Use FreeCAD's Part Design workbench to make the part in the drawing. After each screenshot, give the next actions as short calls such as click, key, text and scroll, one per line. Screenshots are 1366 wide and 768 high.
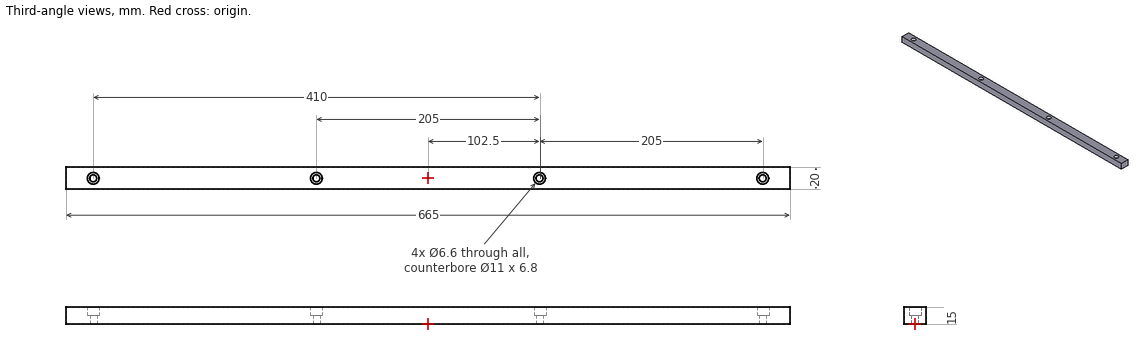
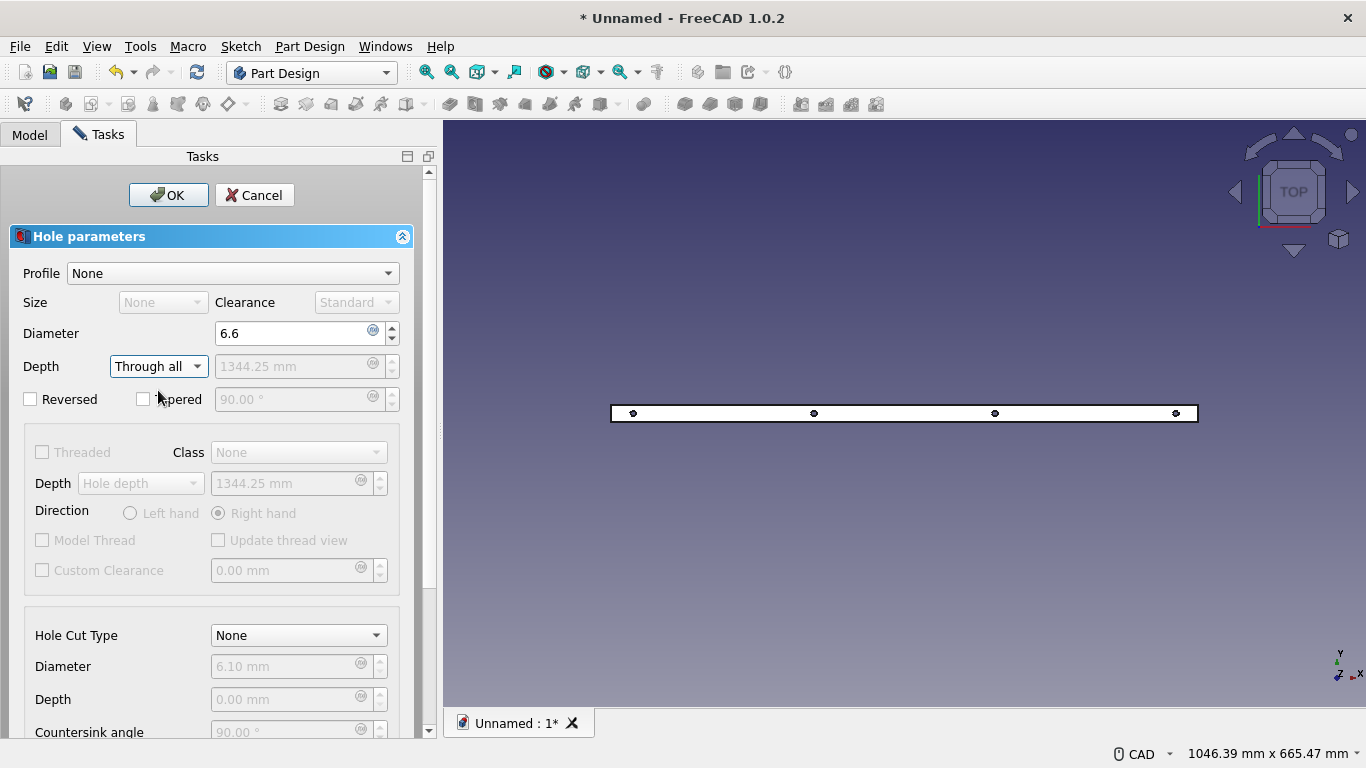
click(300, 636)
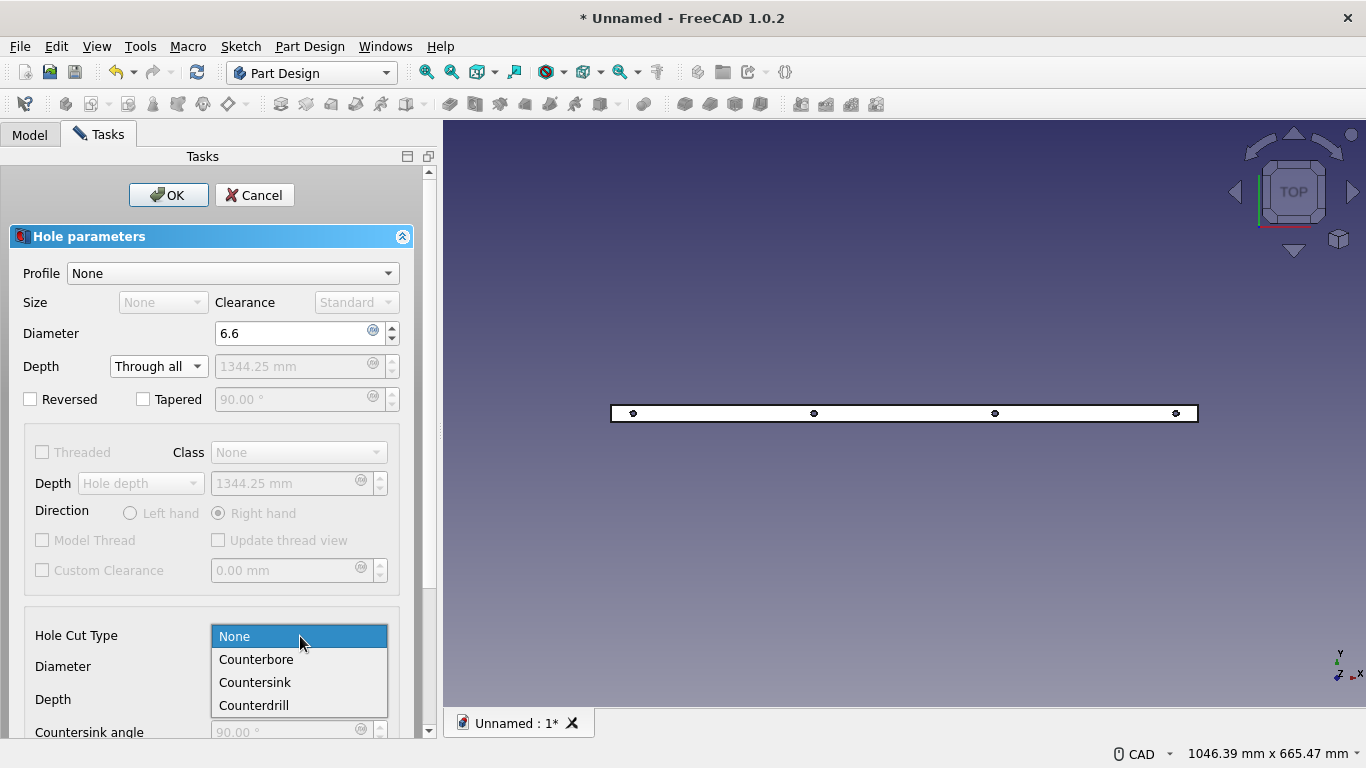
click(298, 660)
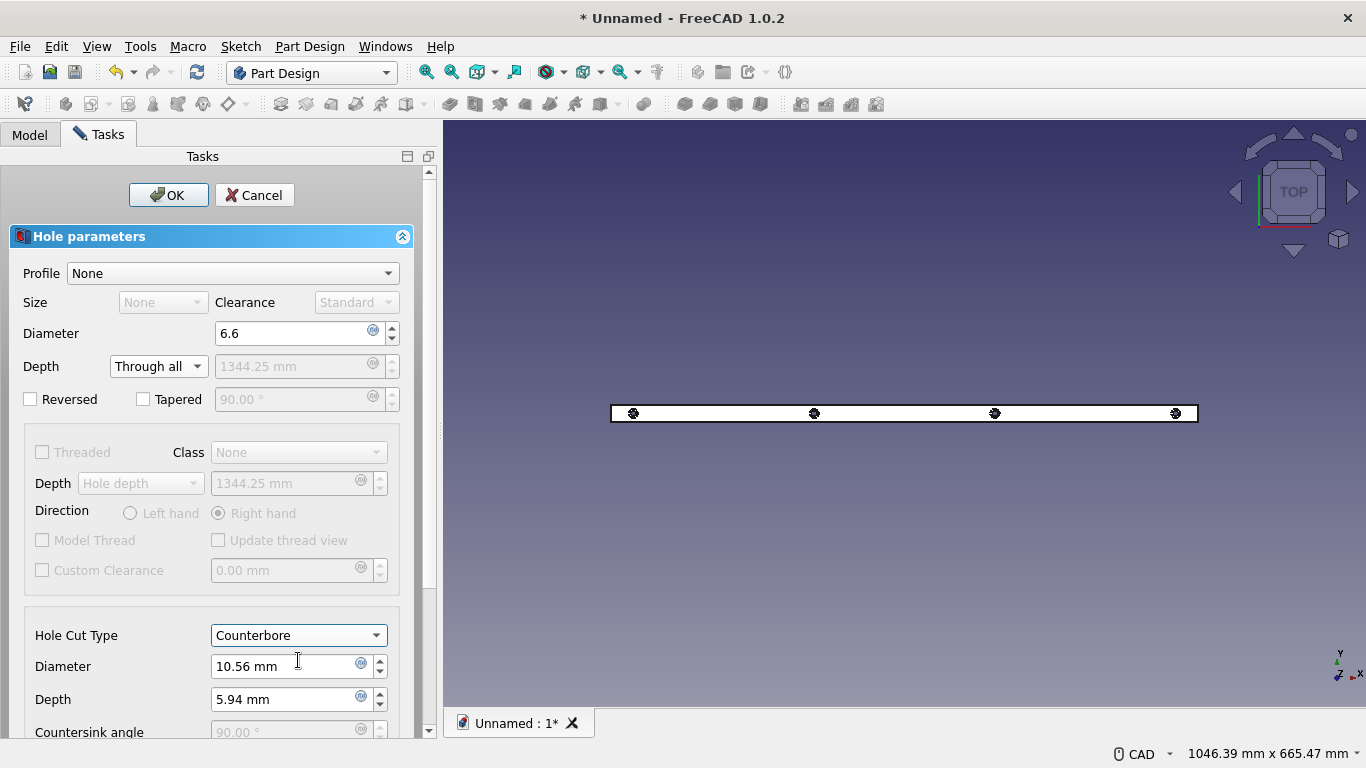
triple_click(292, 666)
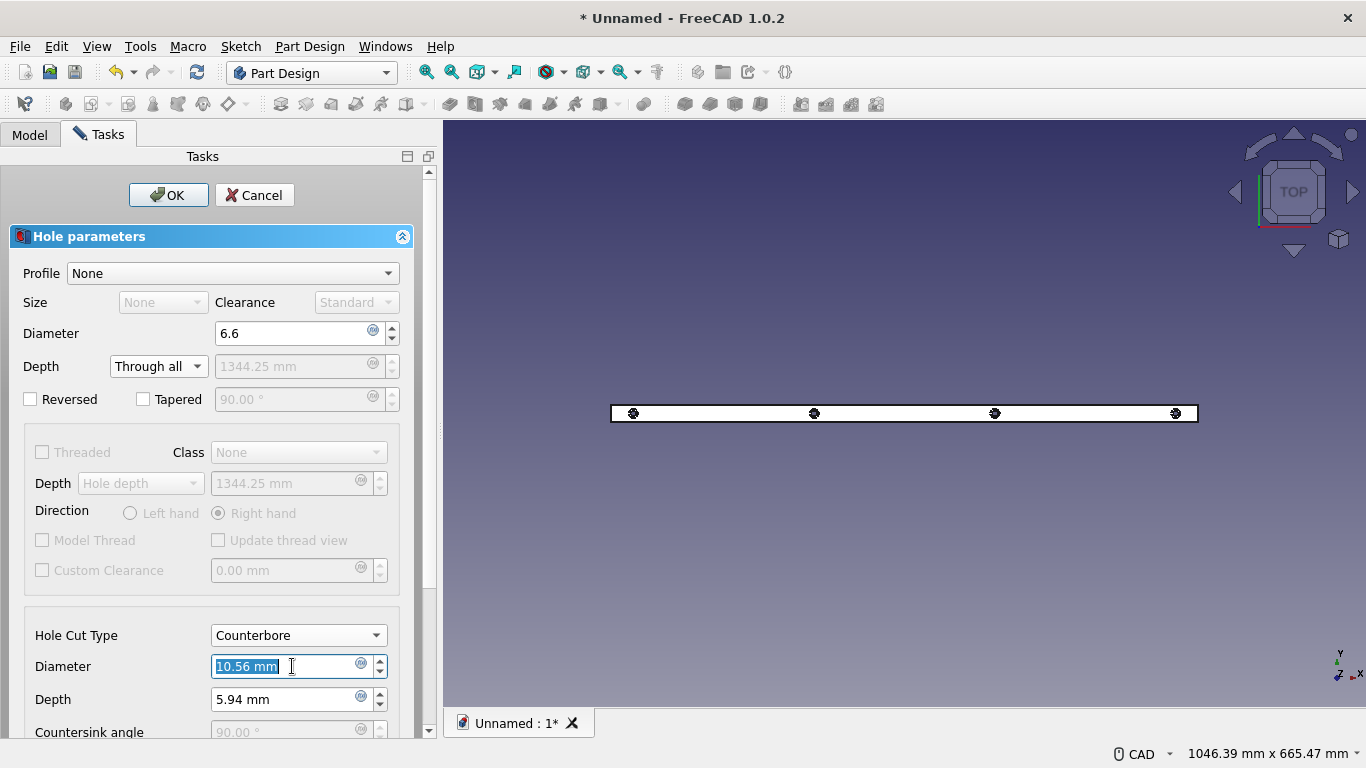
text(11)
key(Tab)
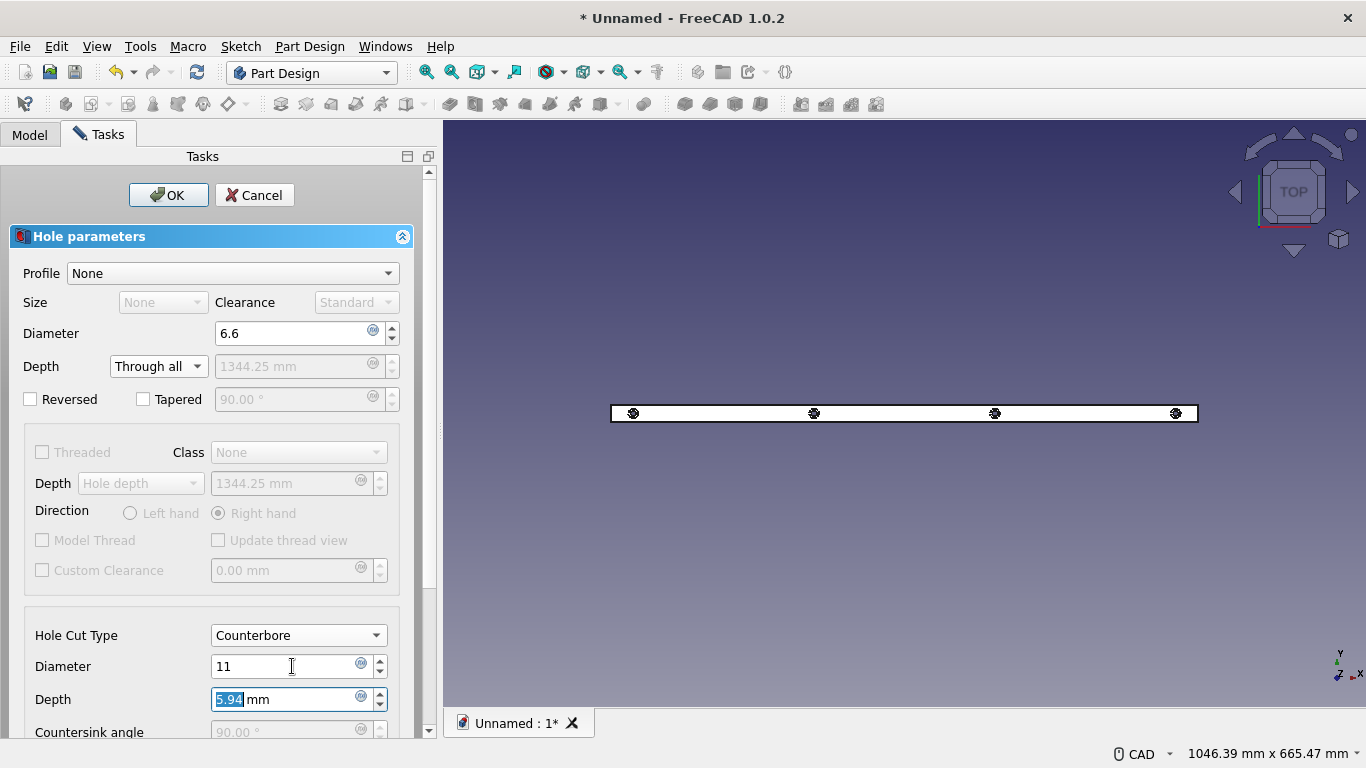
text(6.8)
key(Tab)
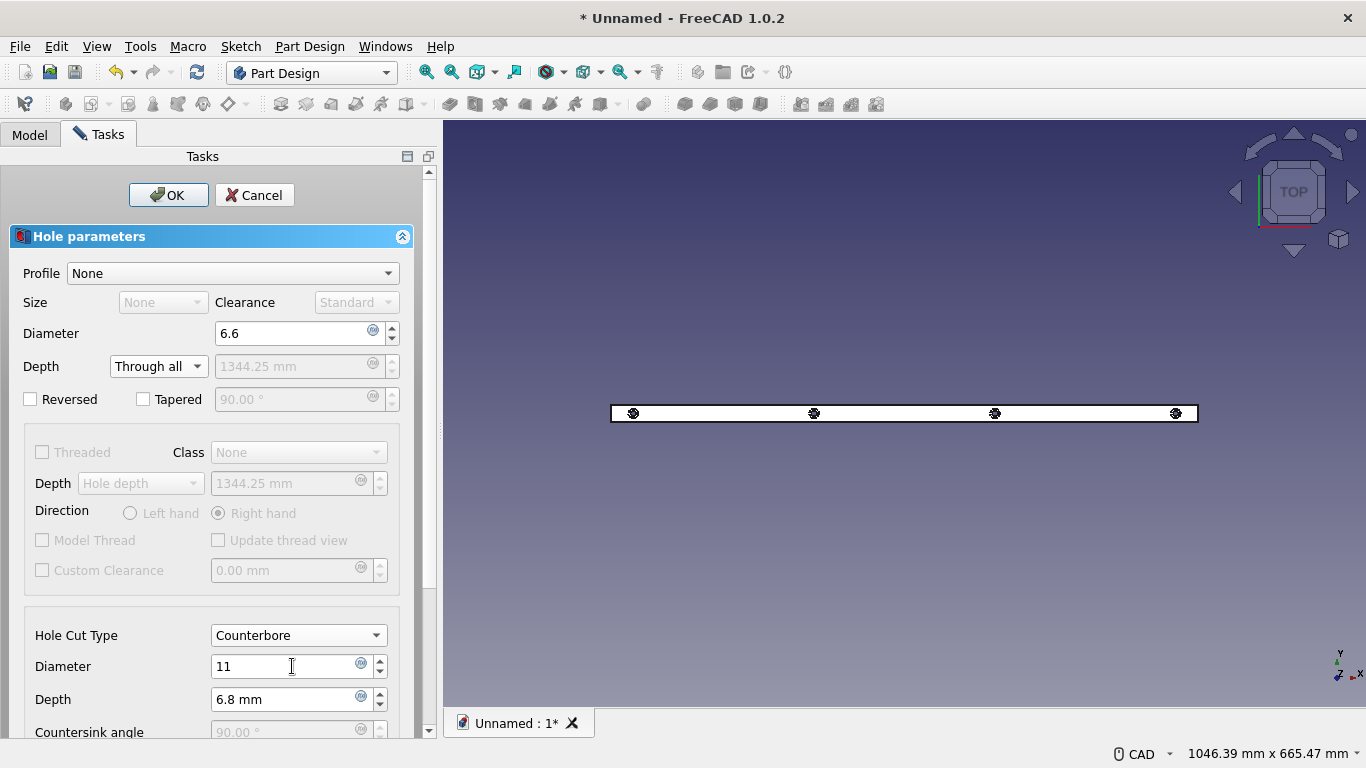
click(169, 195)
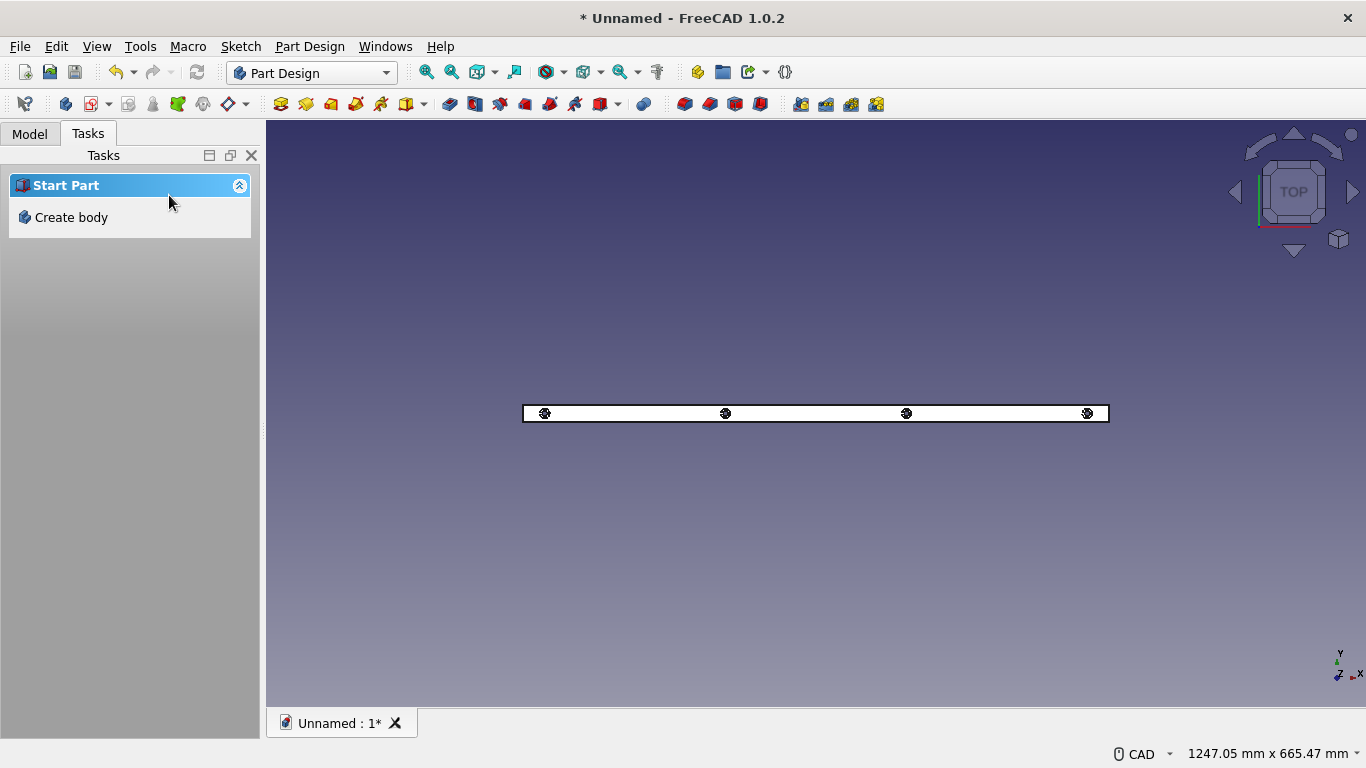
key(0)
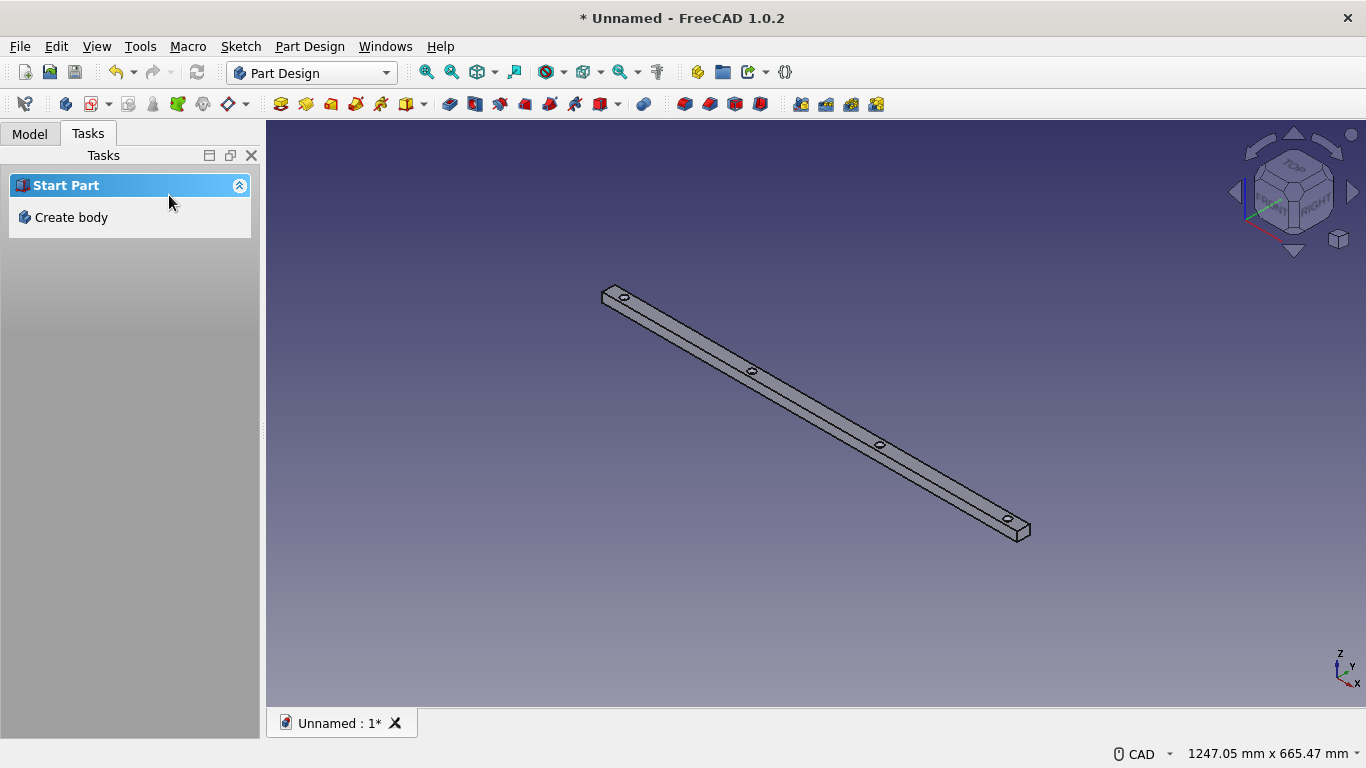
click(427, 72)